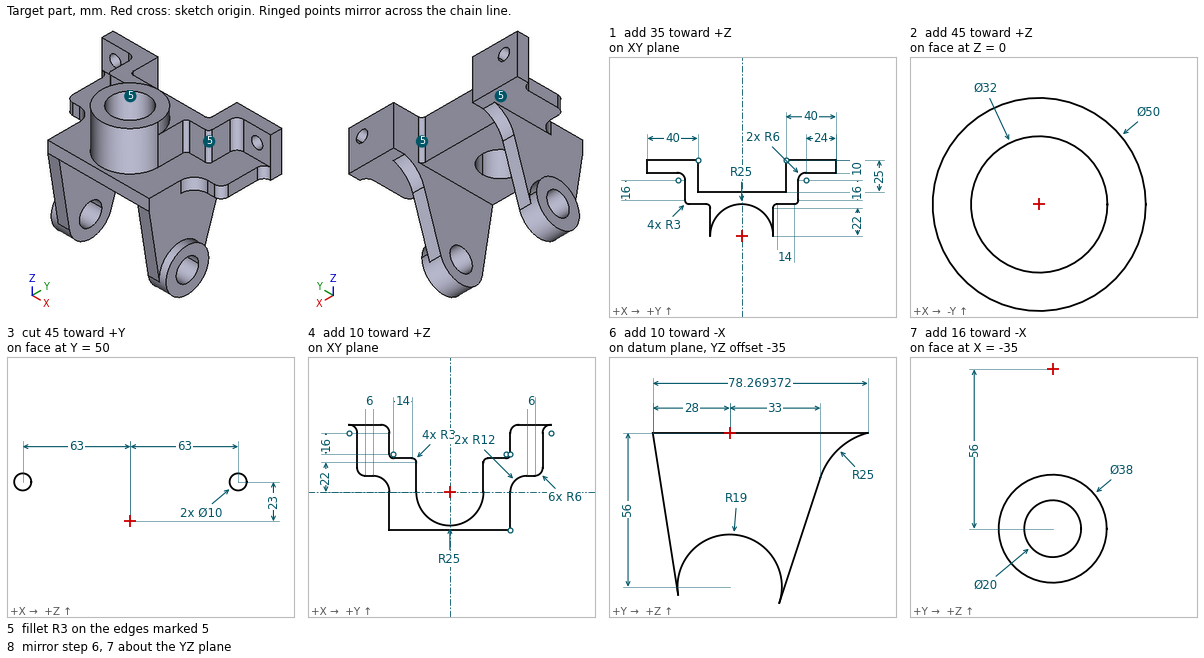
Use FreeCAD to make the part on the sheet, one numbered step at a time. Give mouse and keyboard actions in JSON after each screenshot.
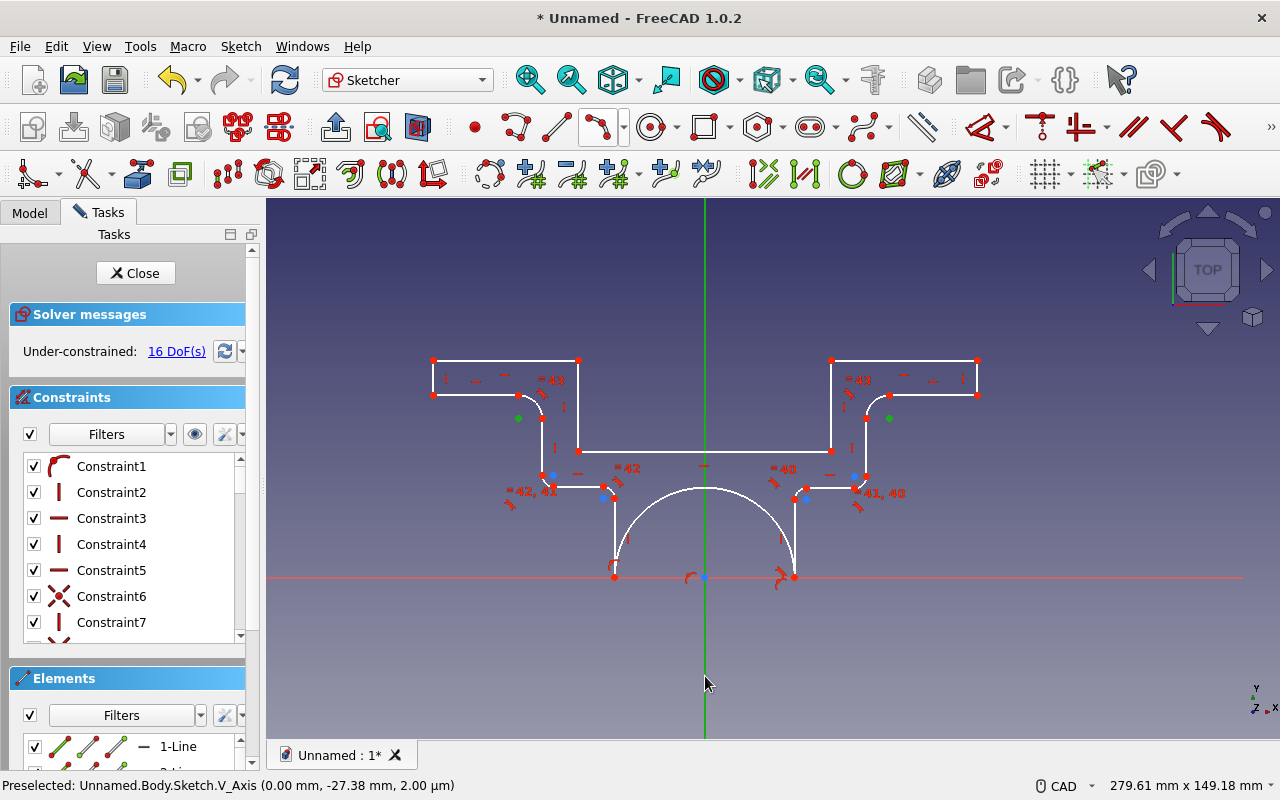
{"action": "key", "text": "s"}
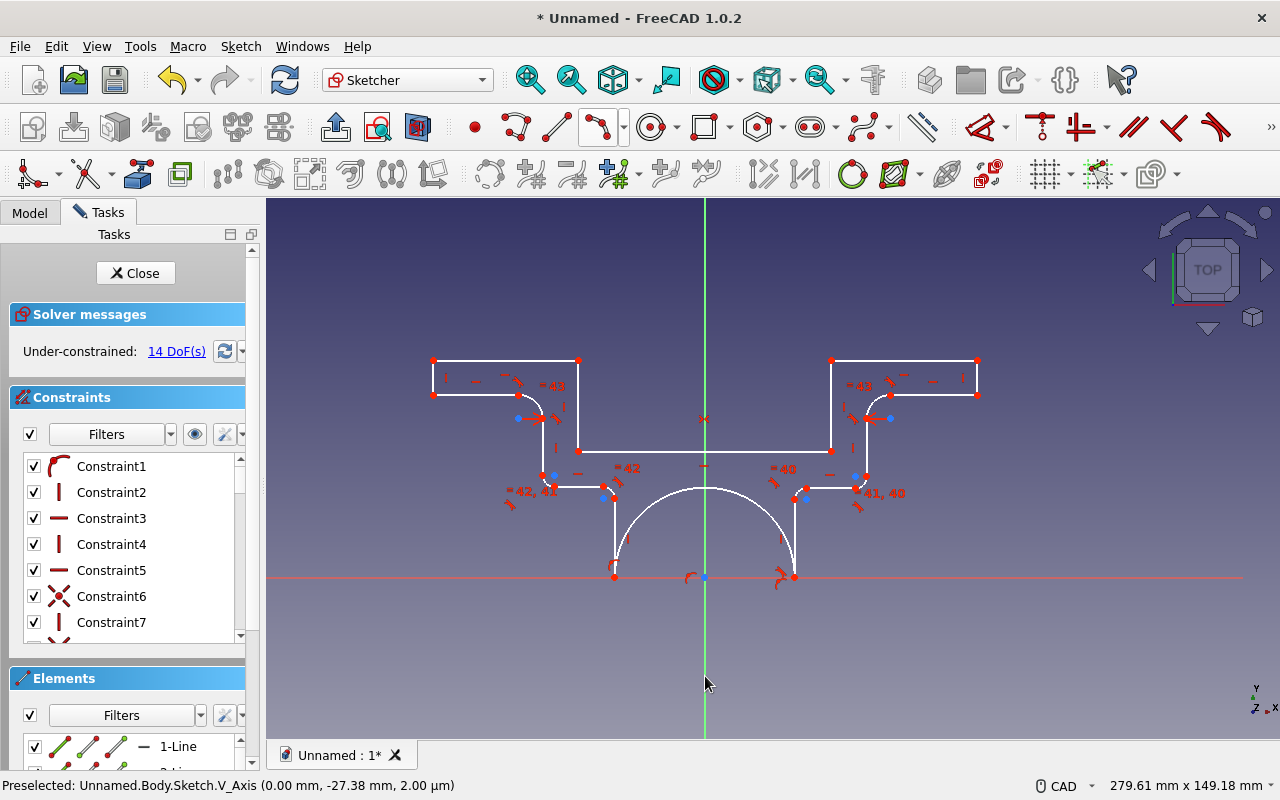
{"action": "left_click", "coordinate": [831, 361]}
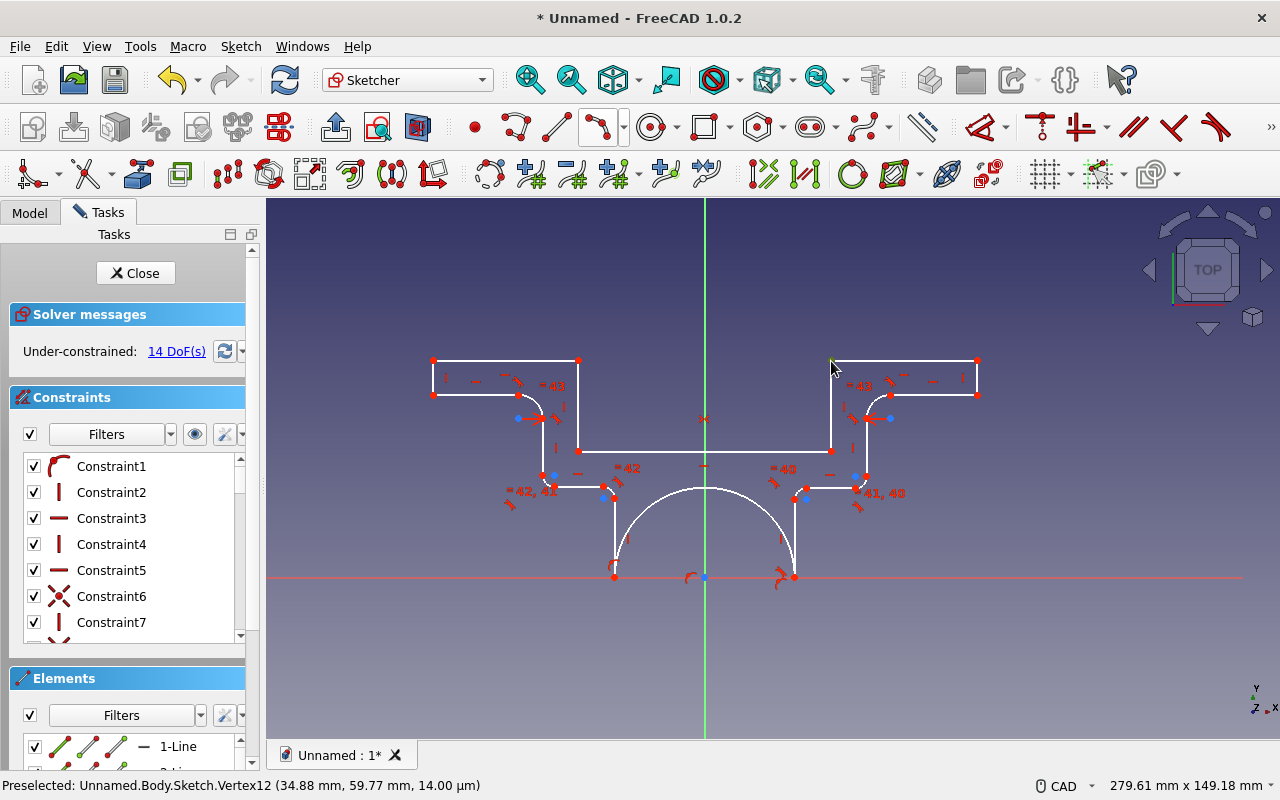
{"action": "left_click", "coordinate": [578, 361]}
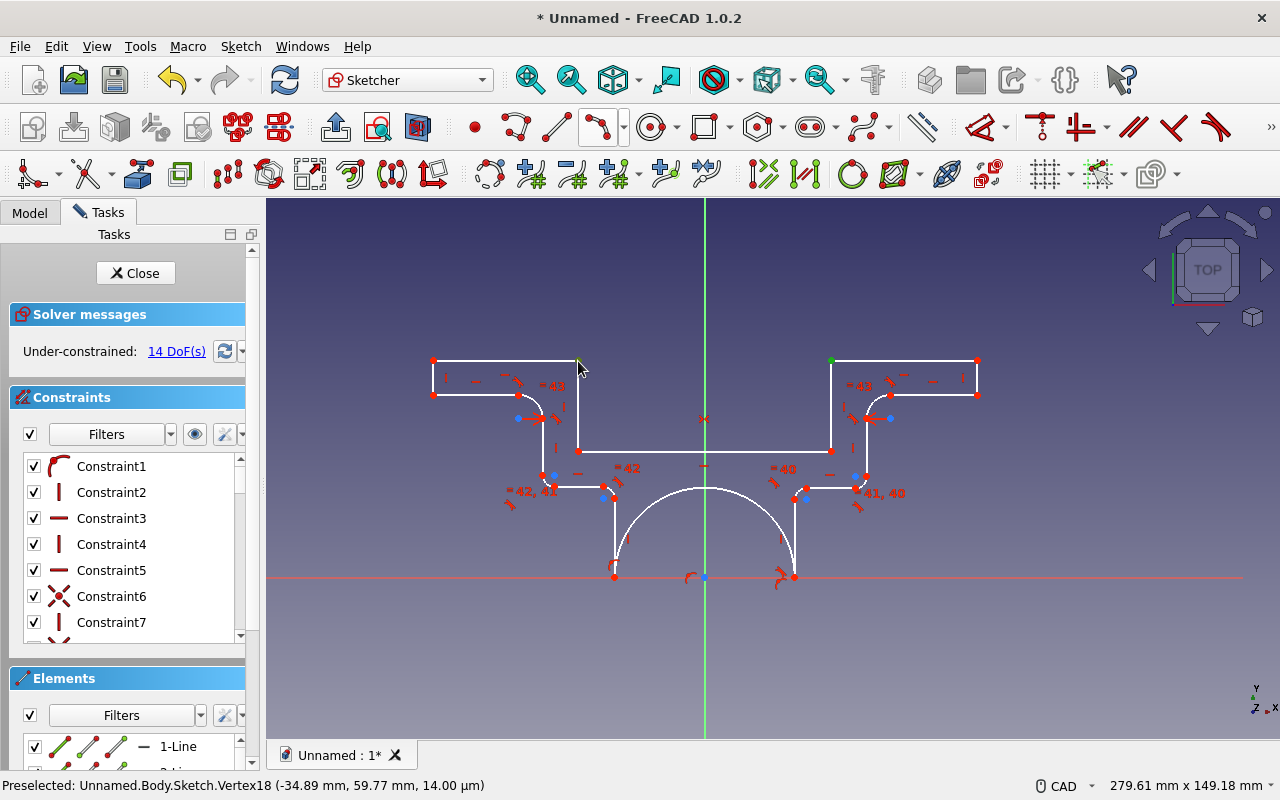
{"action": "left_click", "coordinate": [705, 676]}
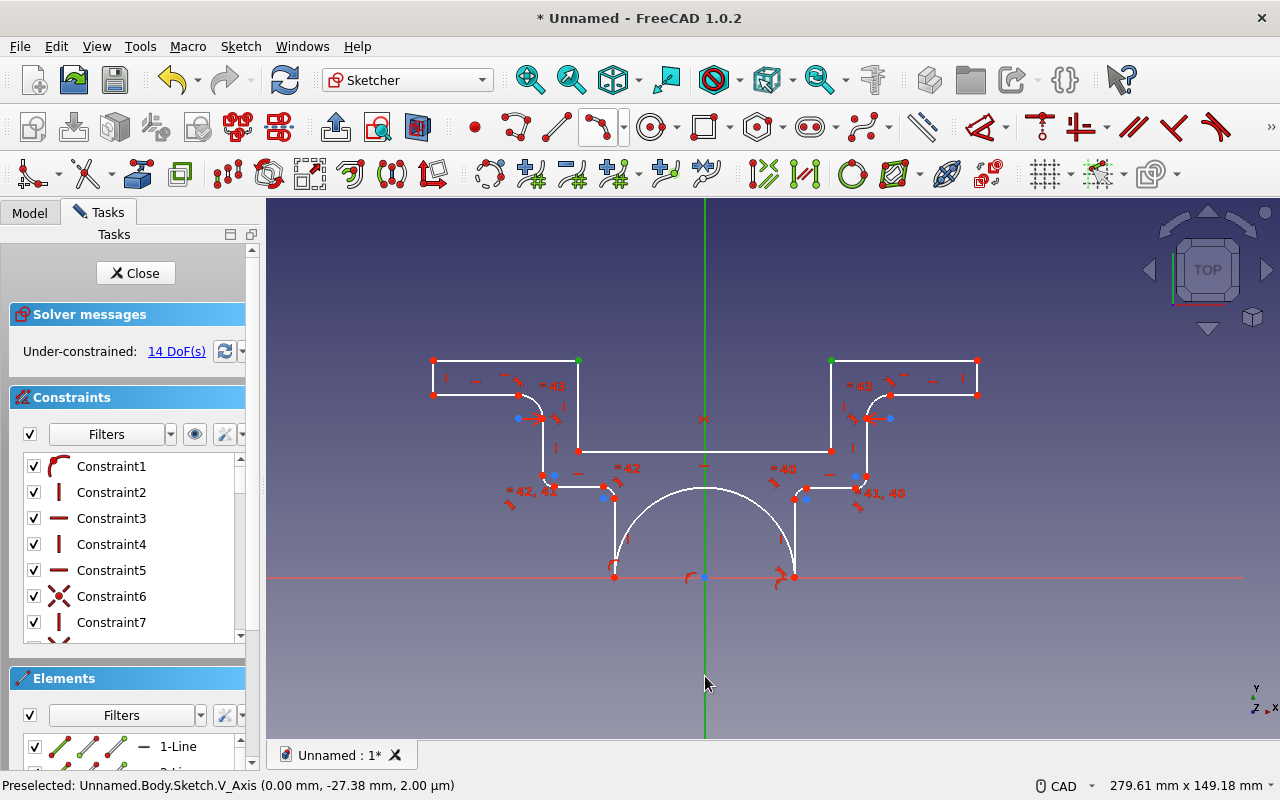
{"action": "key", "text": "s"}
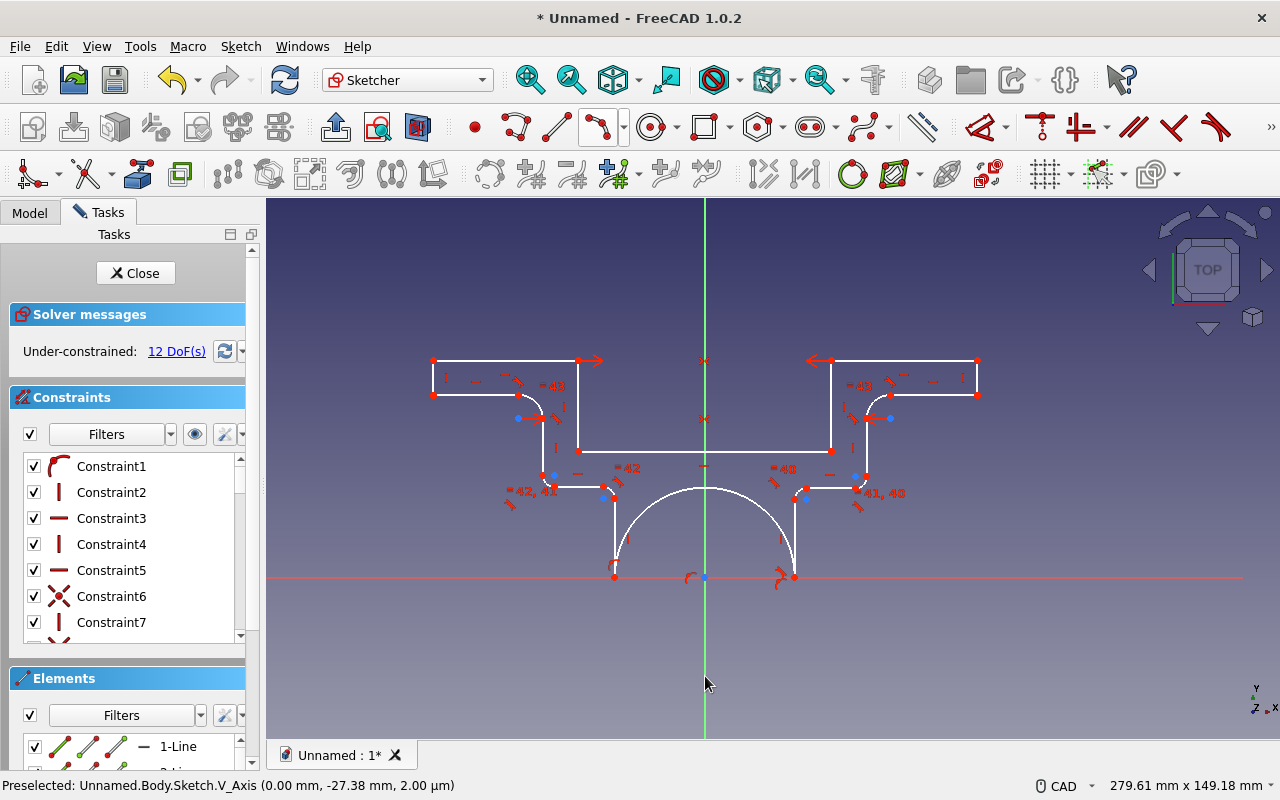
{"action": "left_click", "coordinate": [980, 128]}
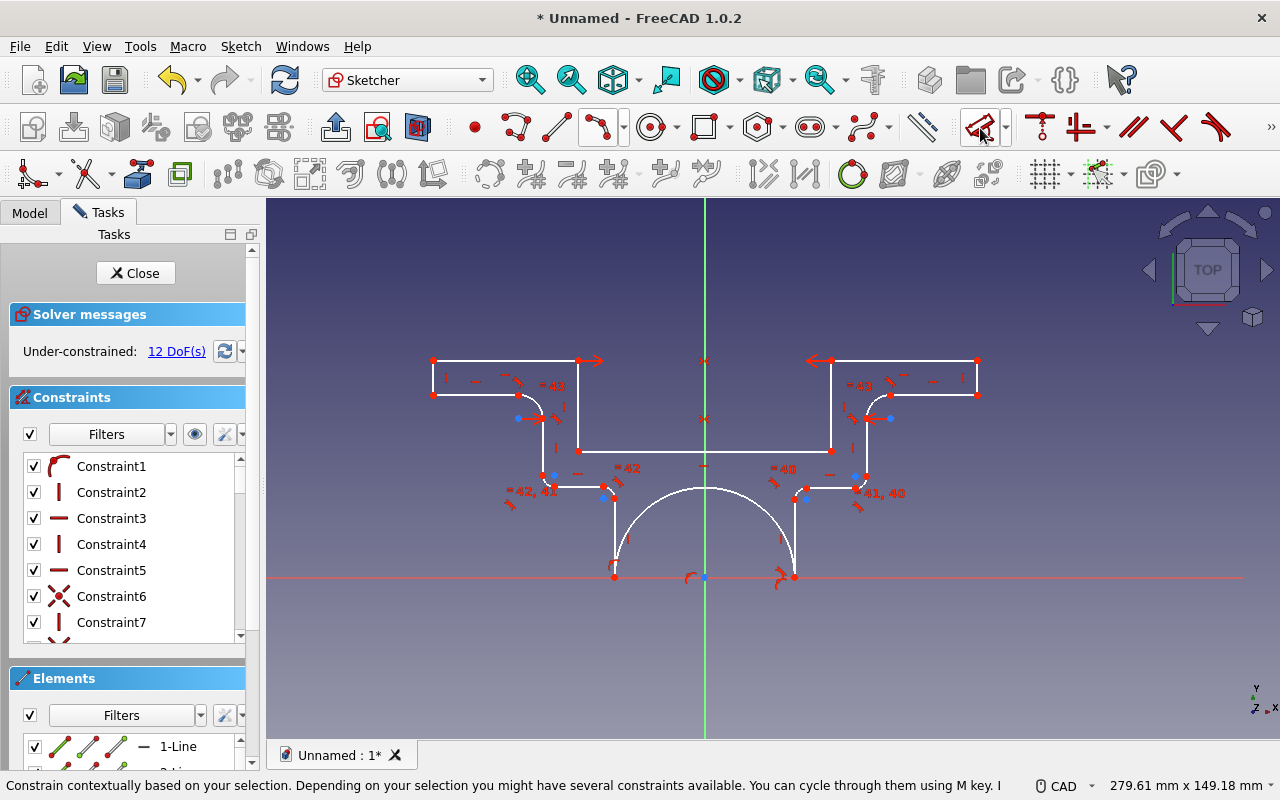
{"action": "scroll", "coordinate": [798, 492], "scroll_direction": "up", "scroll_amount": 7}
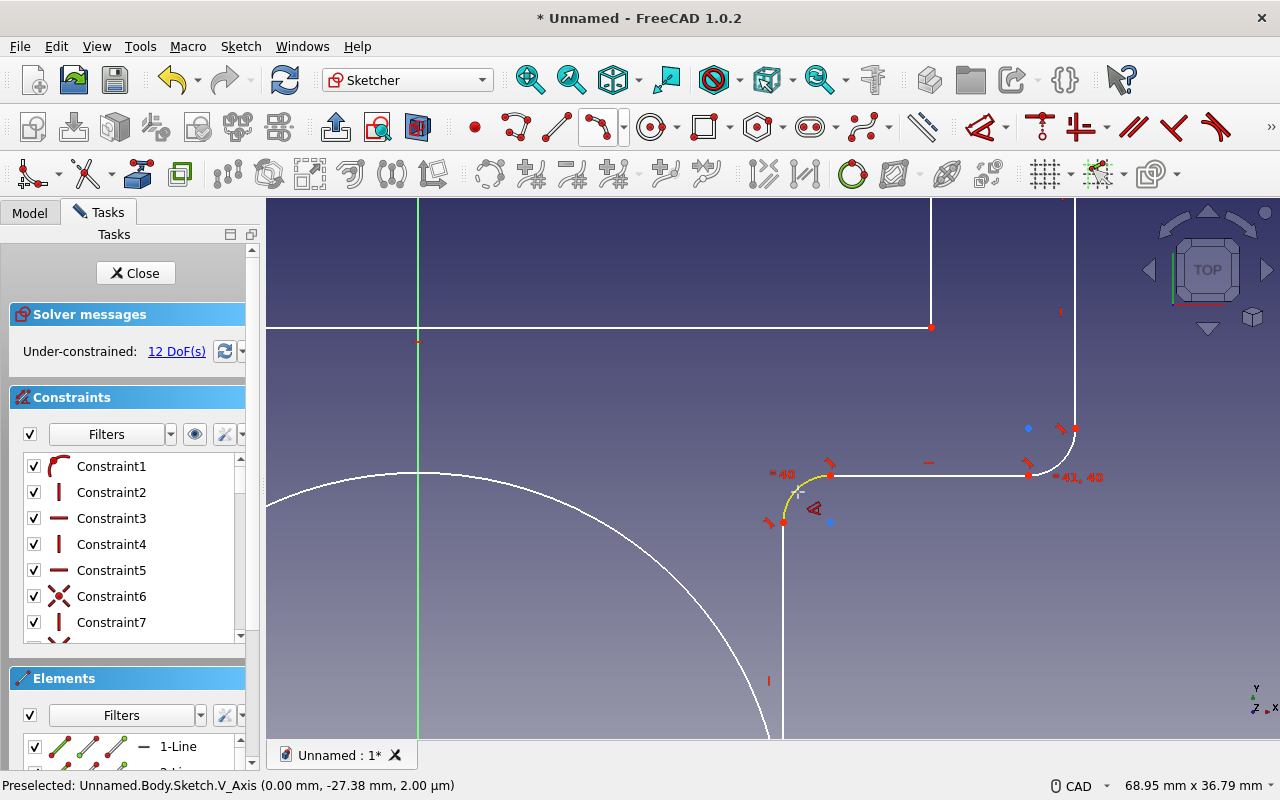
{"action": "left_click", "coordinate": [797, 489]}
{"action": "left_click", "coordinate": [774, 466]}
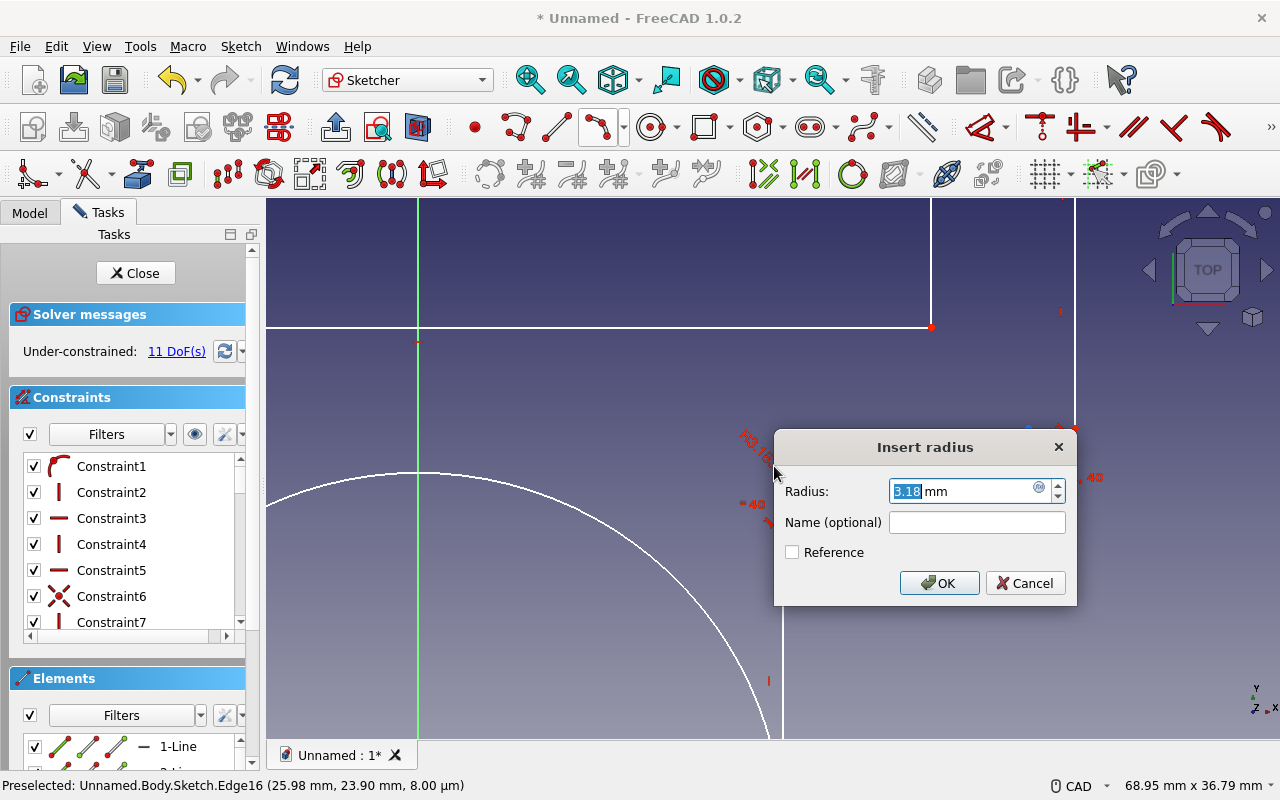
{"action": "type", "text": "3"}
{"action": "key", "text": "Return"}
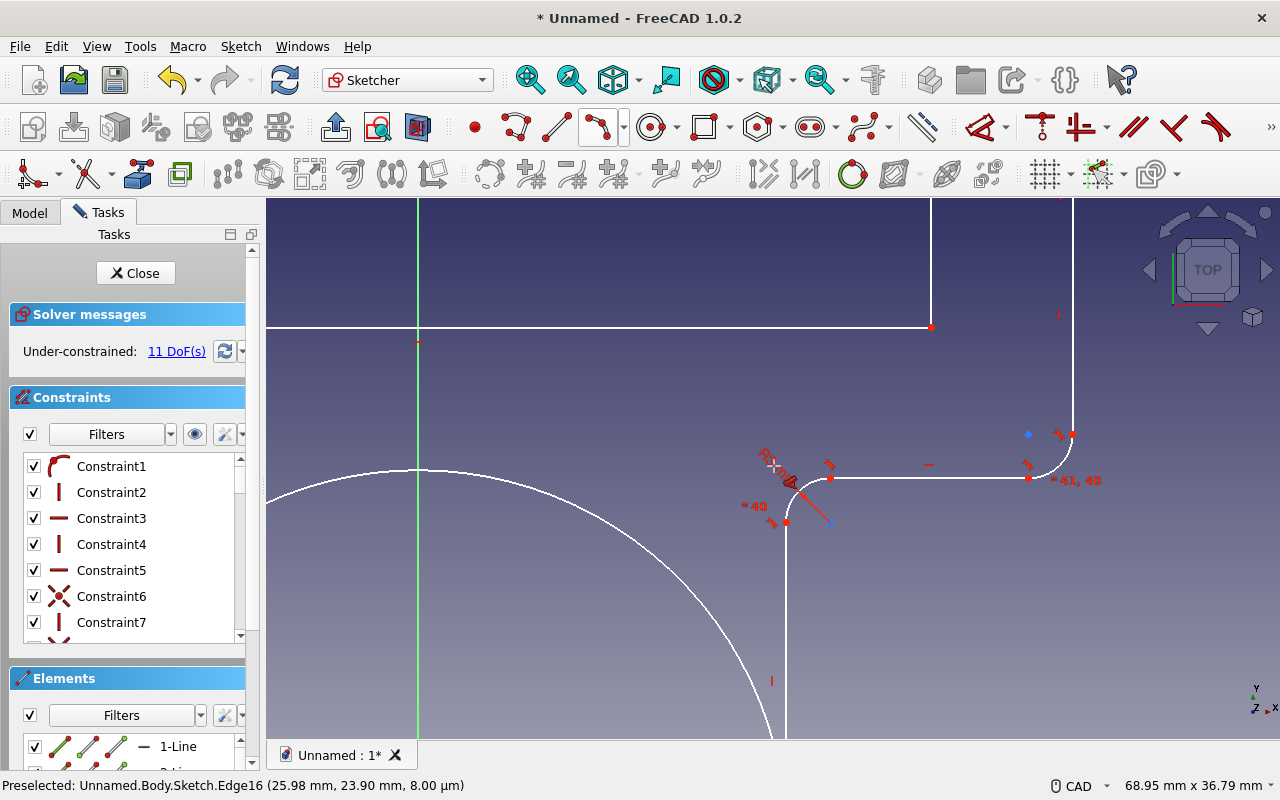
{"action": "scroll", "coordinate": [798, 492], "scroll_direction": "down", "scroll_amount": 7}